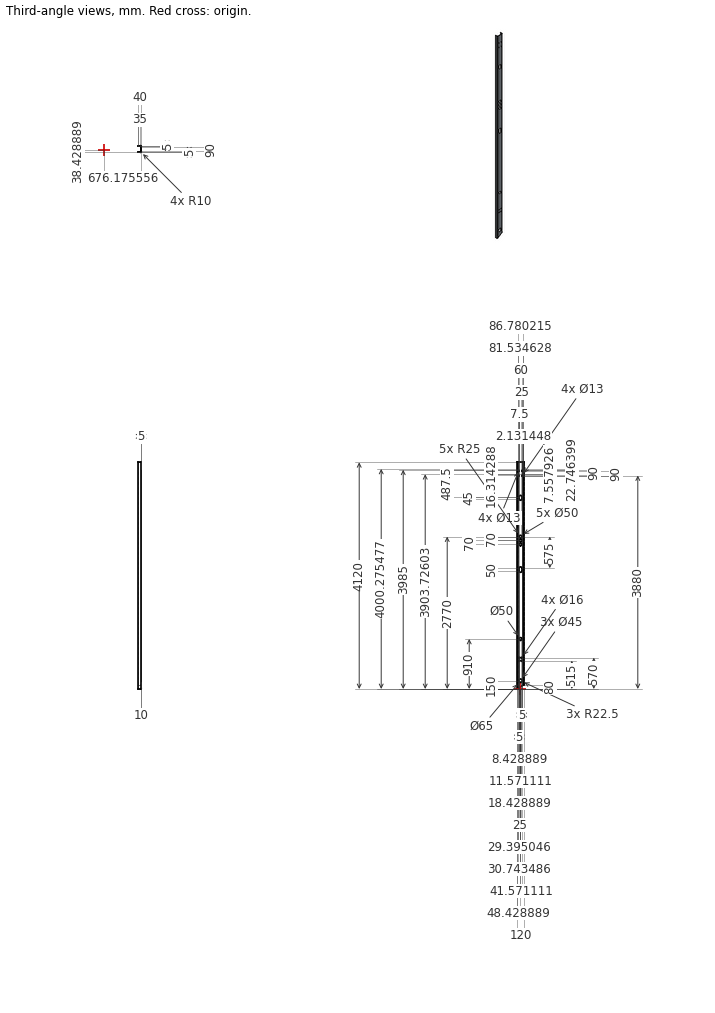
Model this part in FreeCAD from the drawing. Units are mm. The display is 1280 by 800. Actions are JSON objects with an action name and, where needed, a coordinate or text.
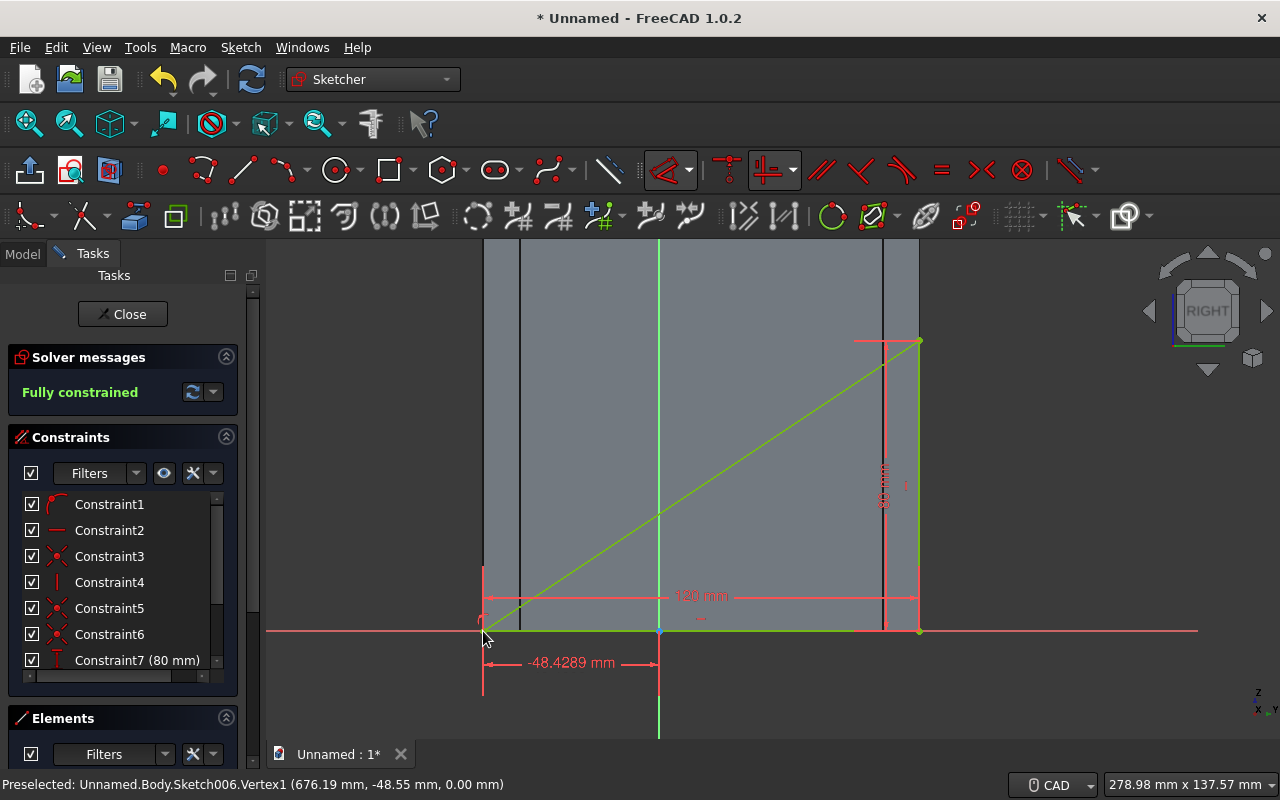
{"action": "left_click", "coordinate": [123, 314]}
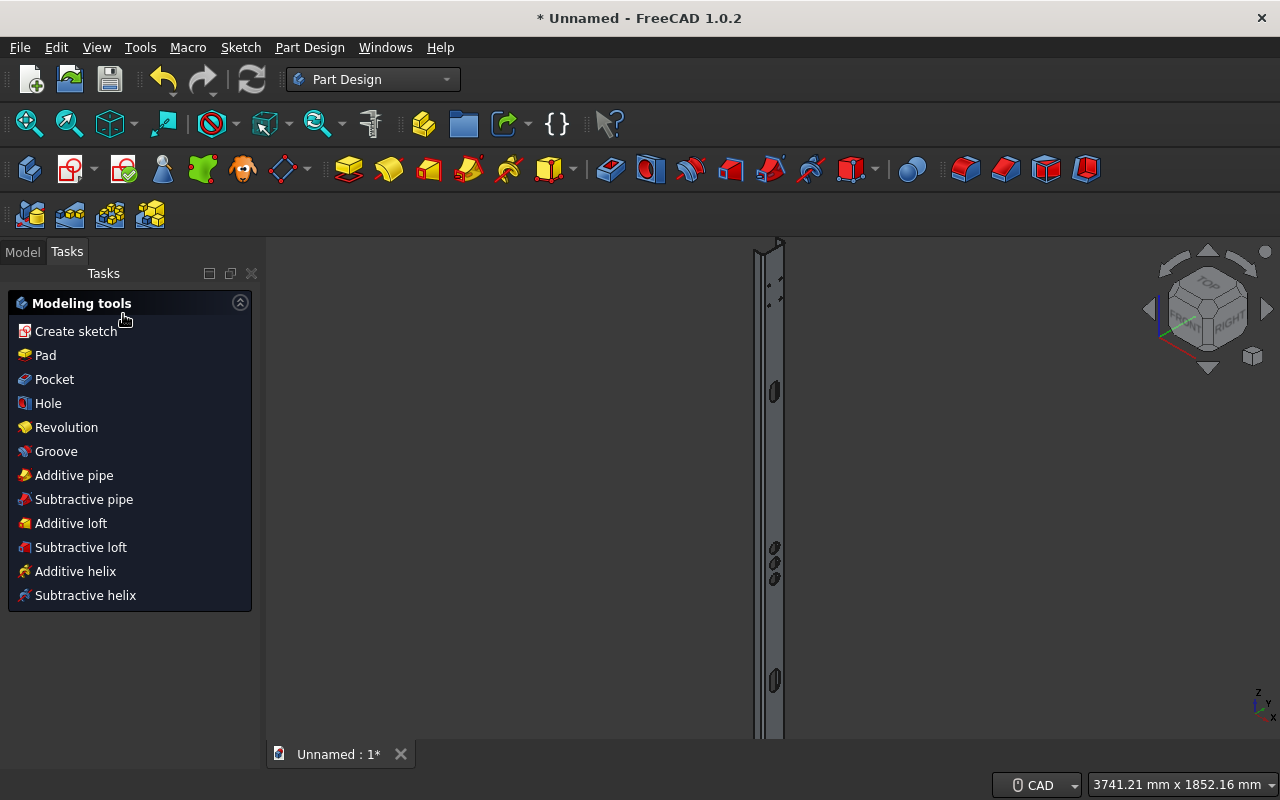
{"action": "left_click", "coordinate": [612, 170]}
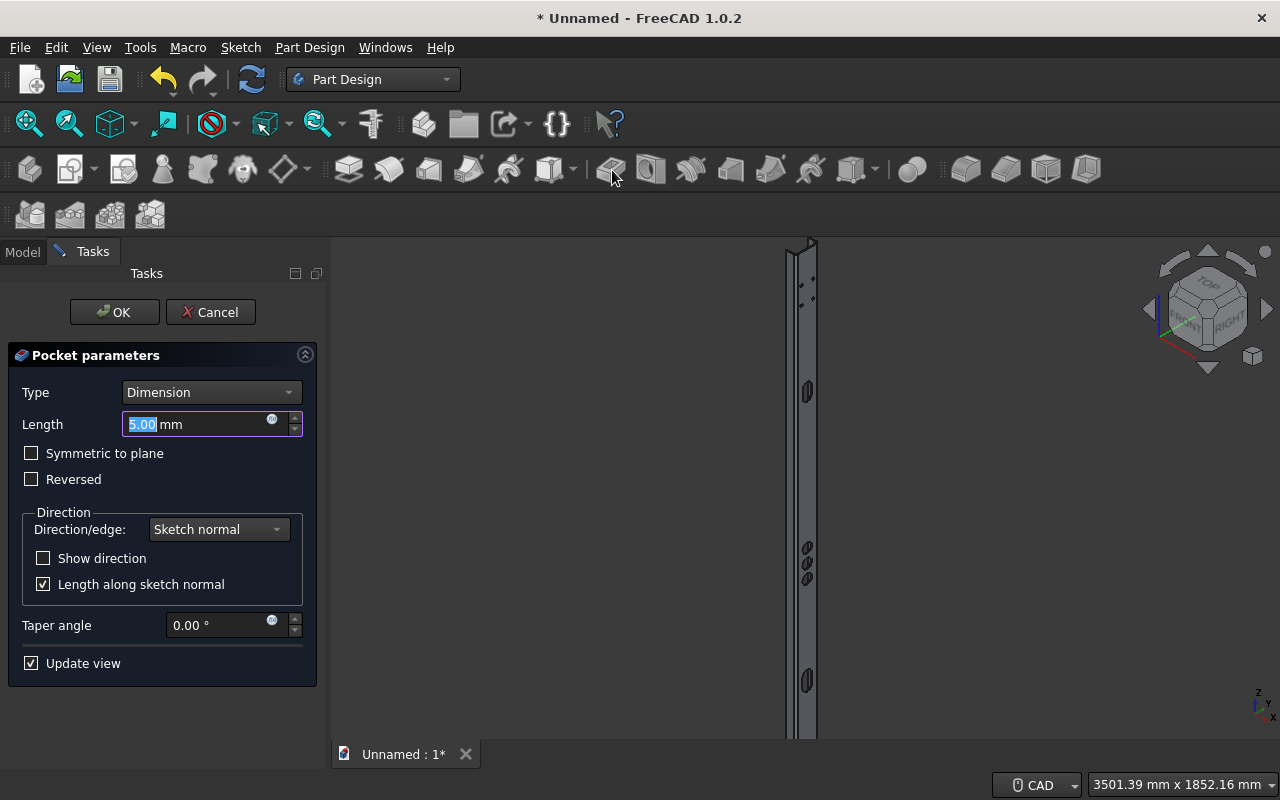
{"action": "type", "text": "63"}
{"action": "key", "text": "Tab"}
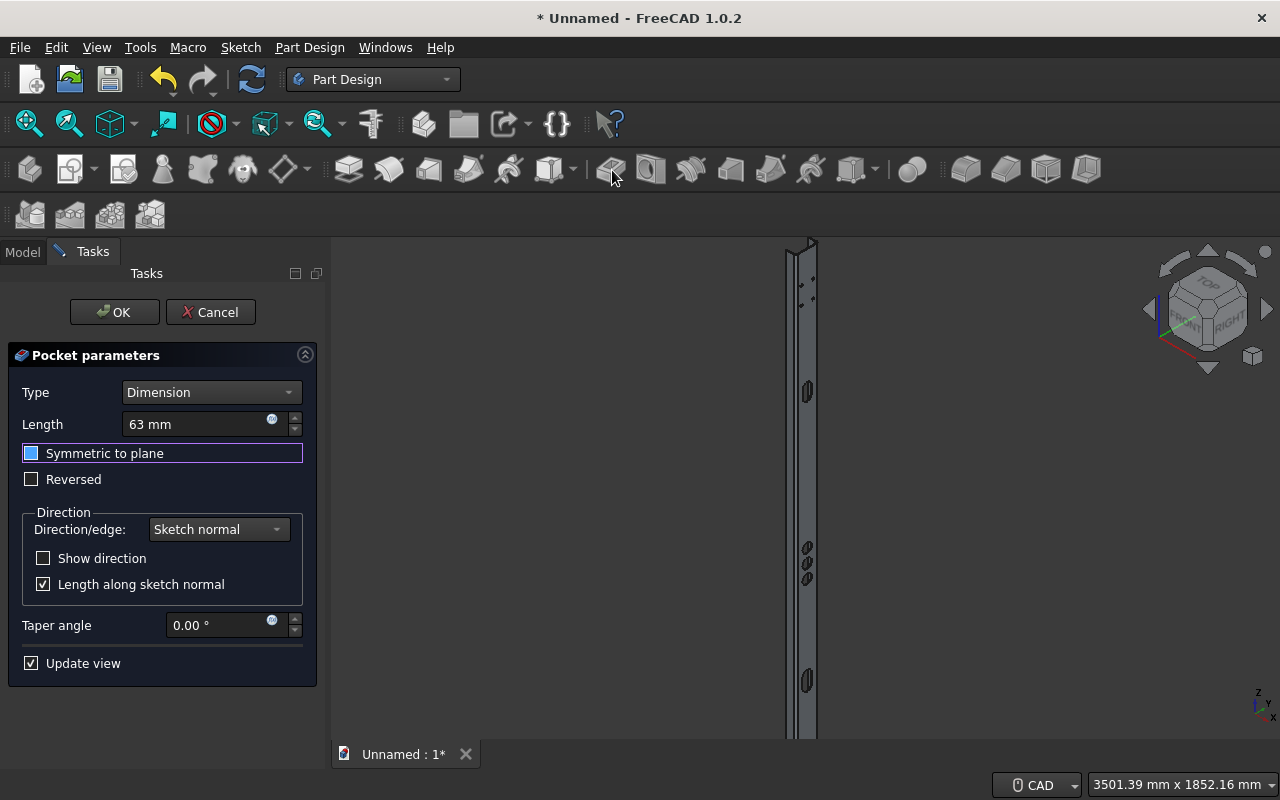
{"action": "left_click", "coordinate": [115, 312]}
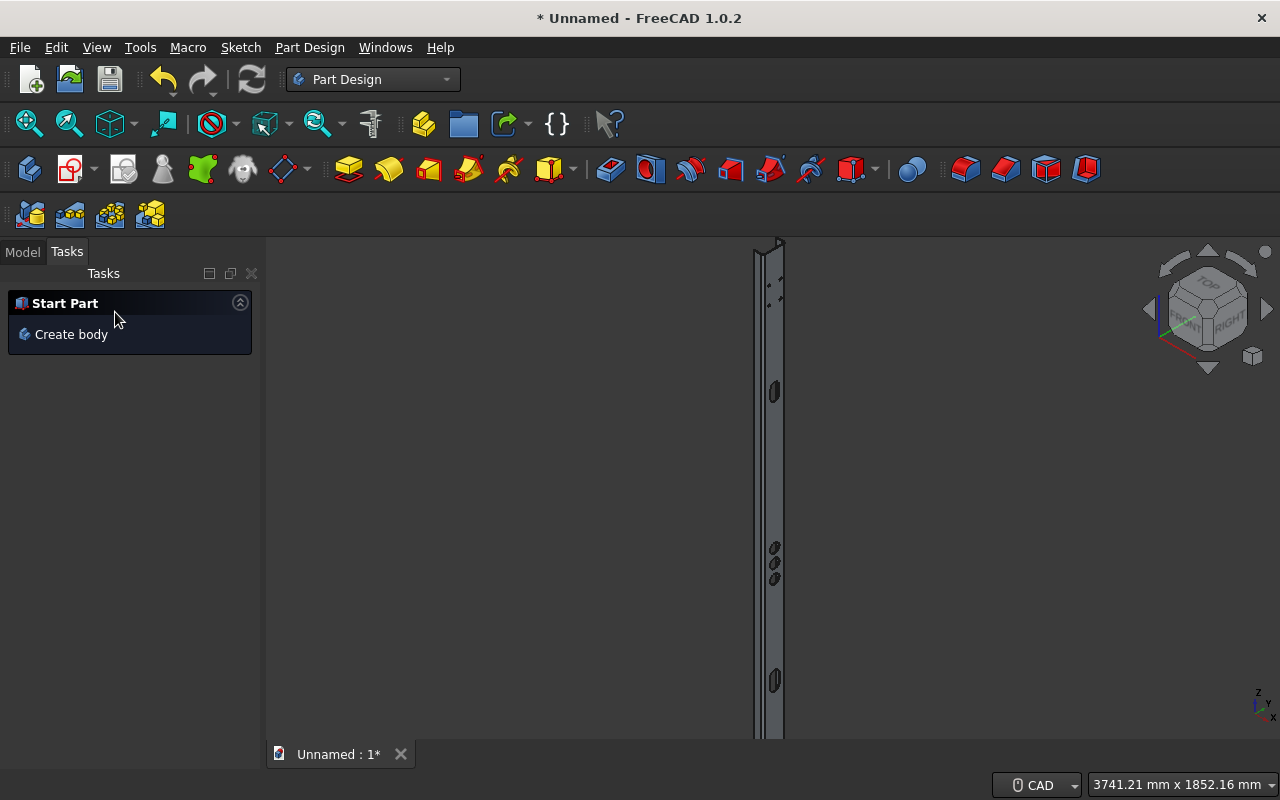
{"action": "key", "text": "v f"}